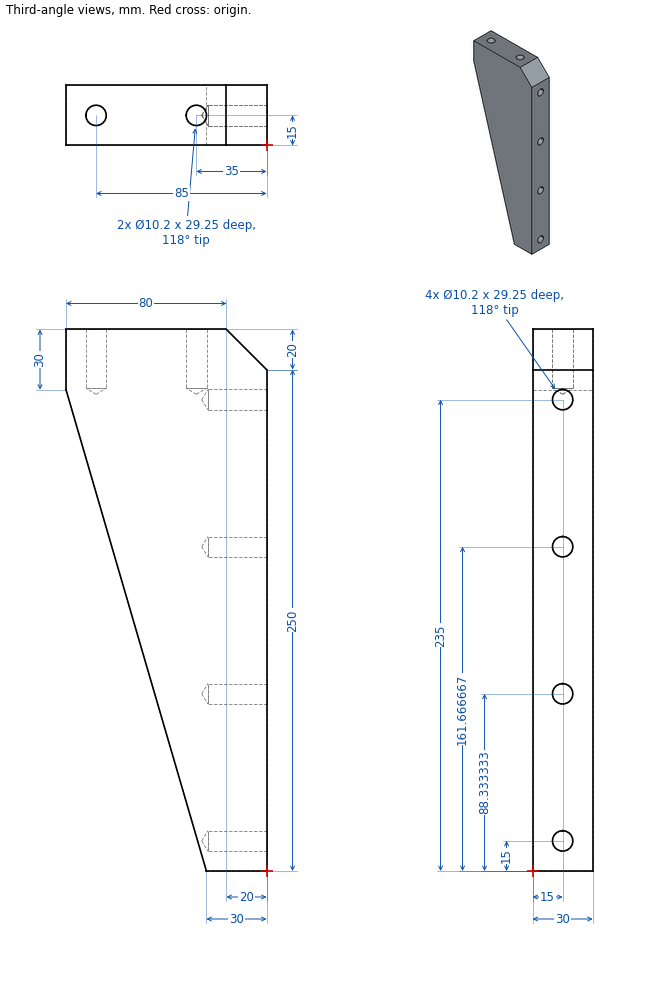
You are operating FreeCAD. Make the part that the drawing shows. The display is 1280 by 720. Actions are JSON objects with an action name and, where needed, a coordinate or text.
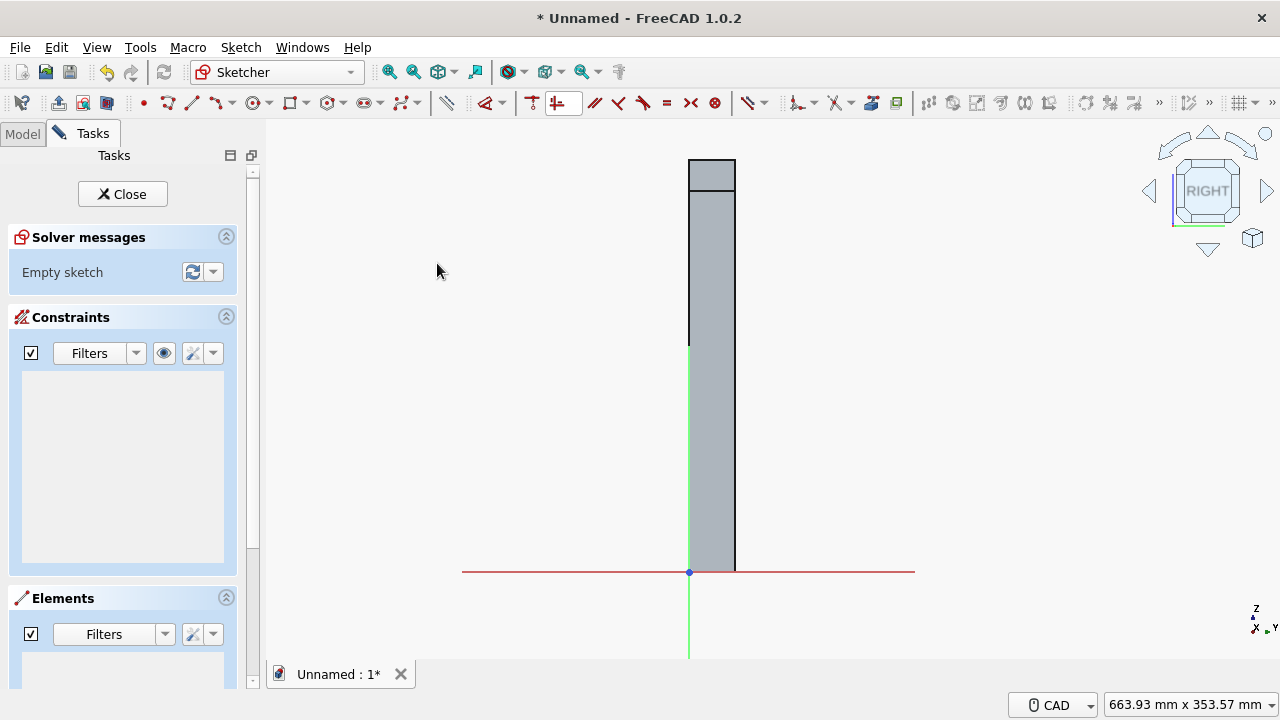
{"action": "key", "text": "g c"}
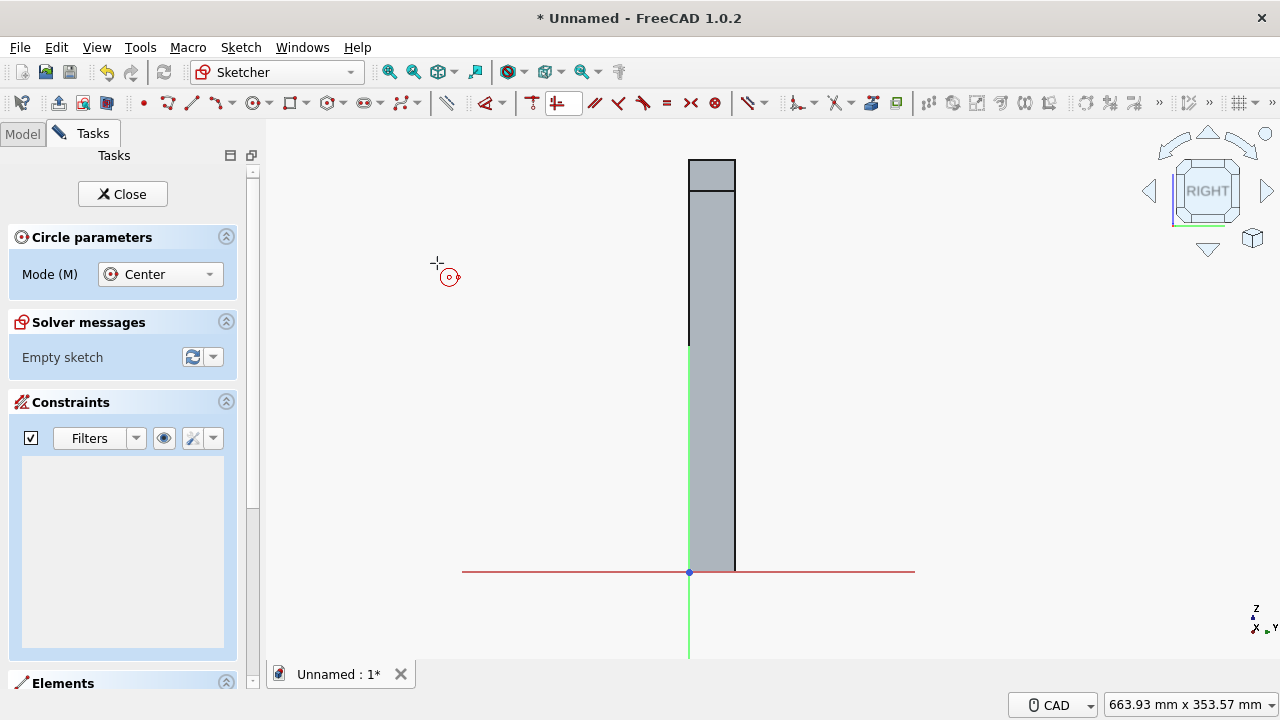
{"action": "scroll", "coordinate": [712, 213], "scroll_direction": "up", "scroll_amount": 6}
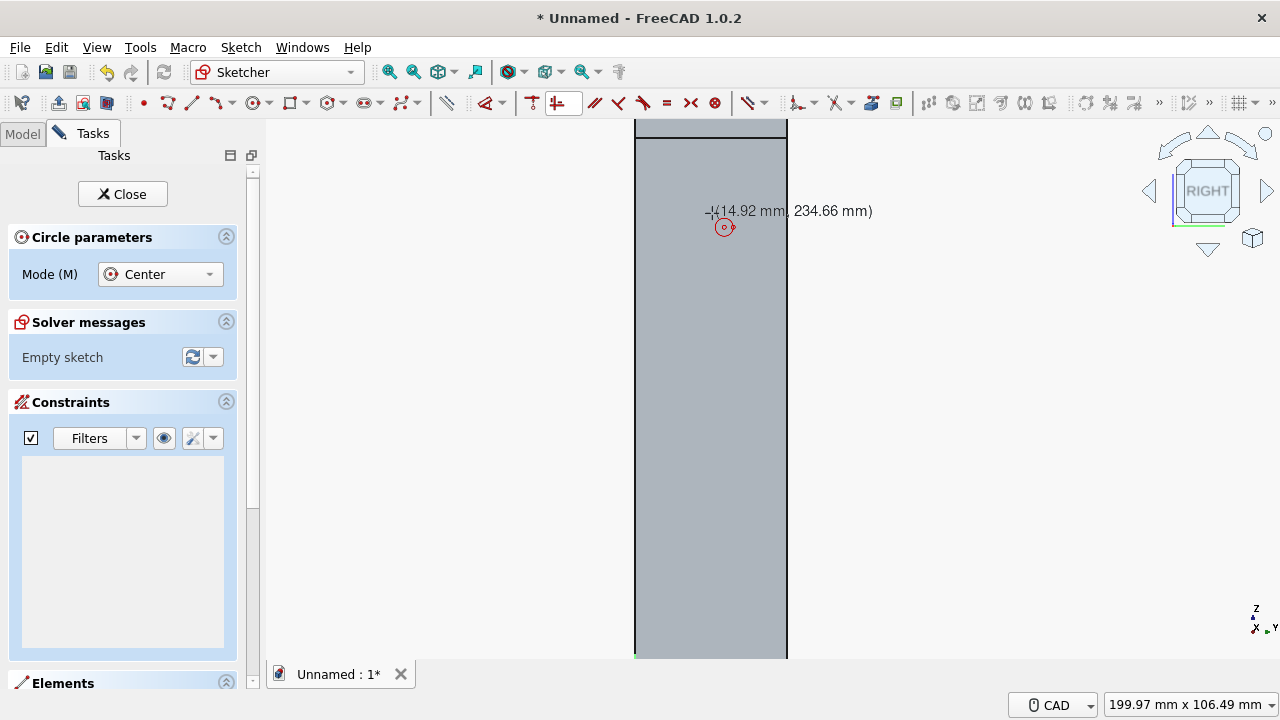
{"action": "left_click", "coordinate": [711, 214]}
{"action": "left_click", "coordinate": [730, 196]}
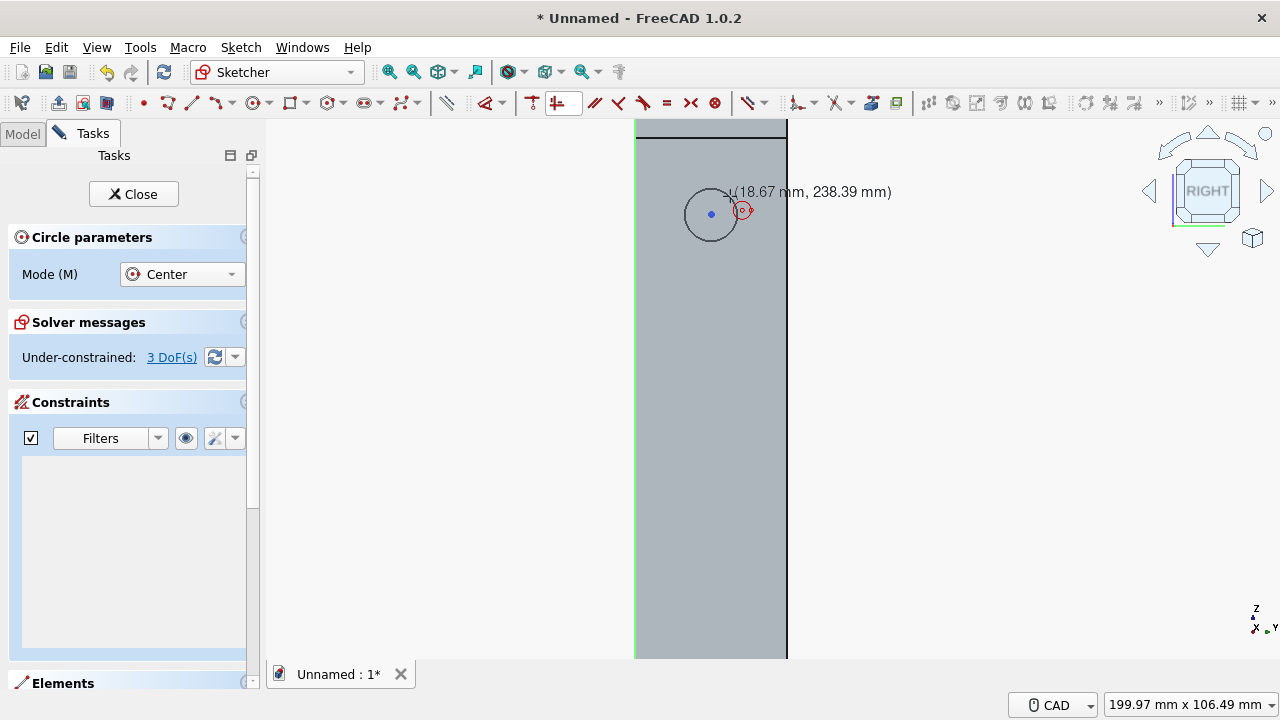
{"action": "scroll", "coordinate": [712, 213], "scroll_direction": "down", "scroll_amount": 6}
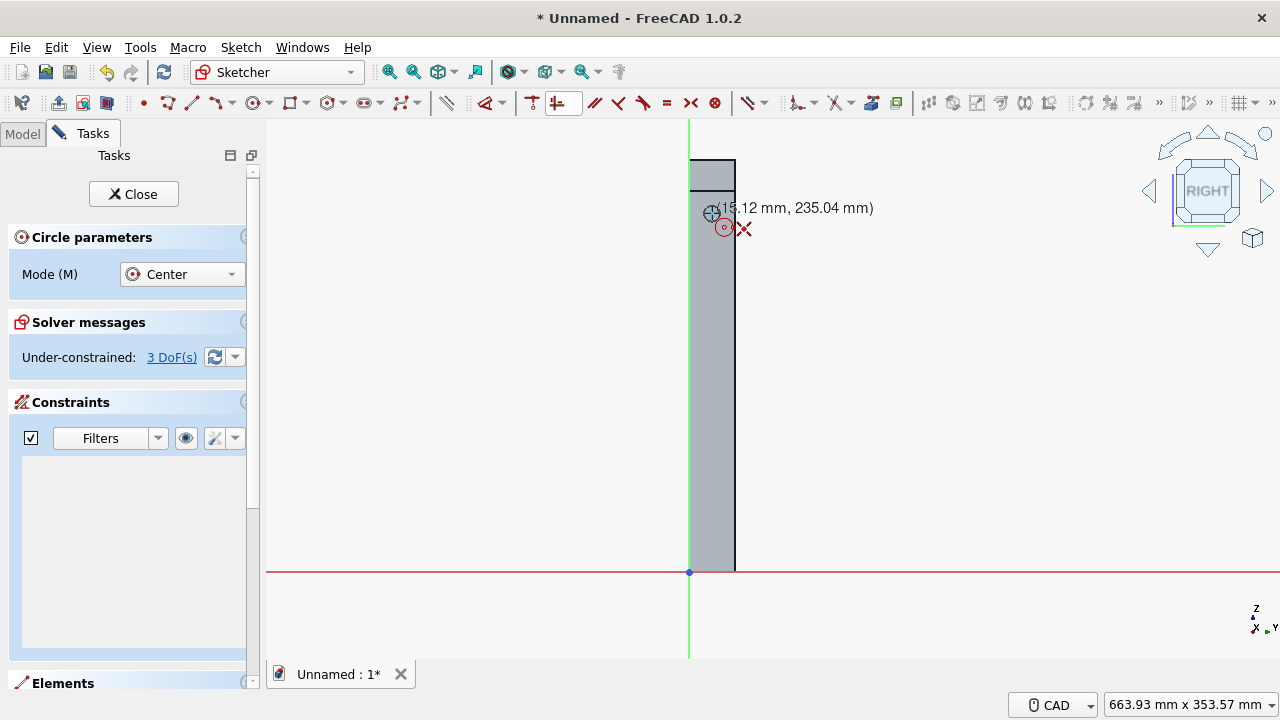
{"action": "scroll", "coordinate": [712, 549], "scroll_direction": "up", "scroll_amount": 6}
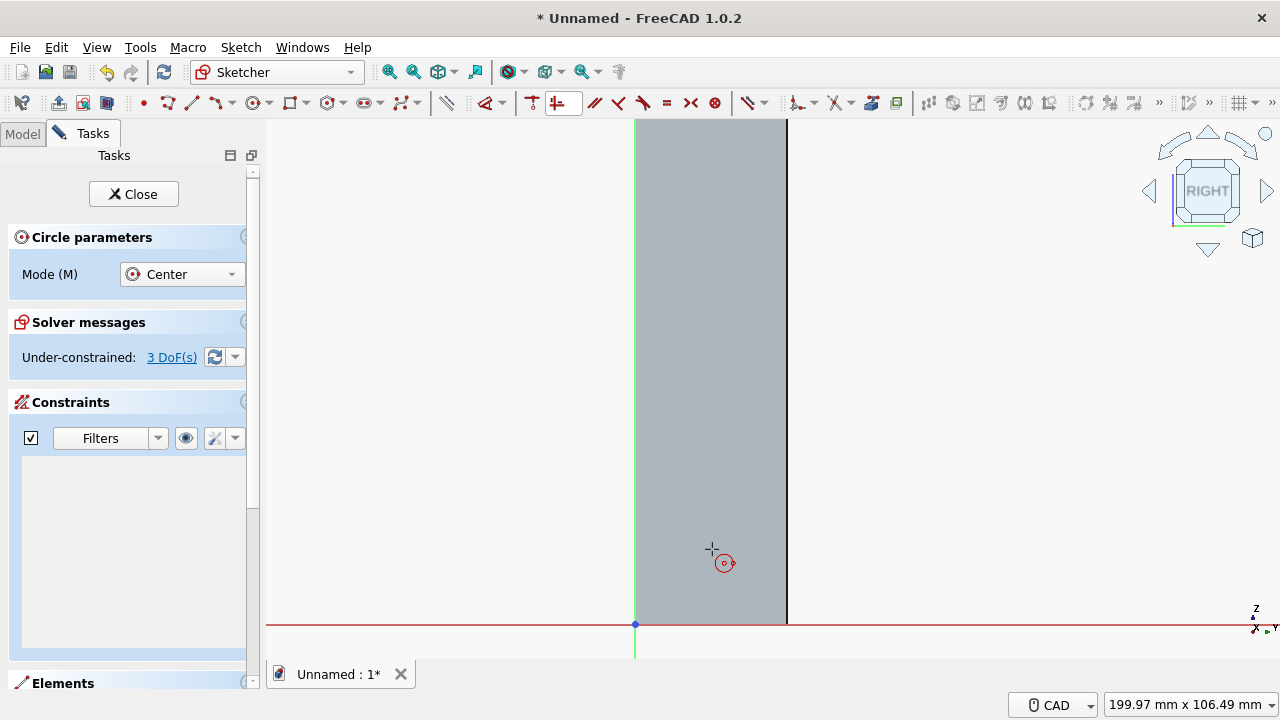
{"action": "left_click", "coordinate": [711, 549]}
{"action": "left_click", "coordinate": [730, 530]}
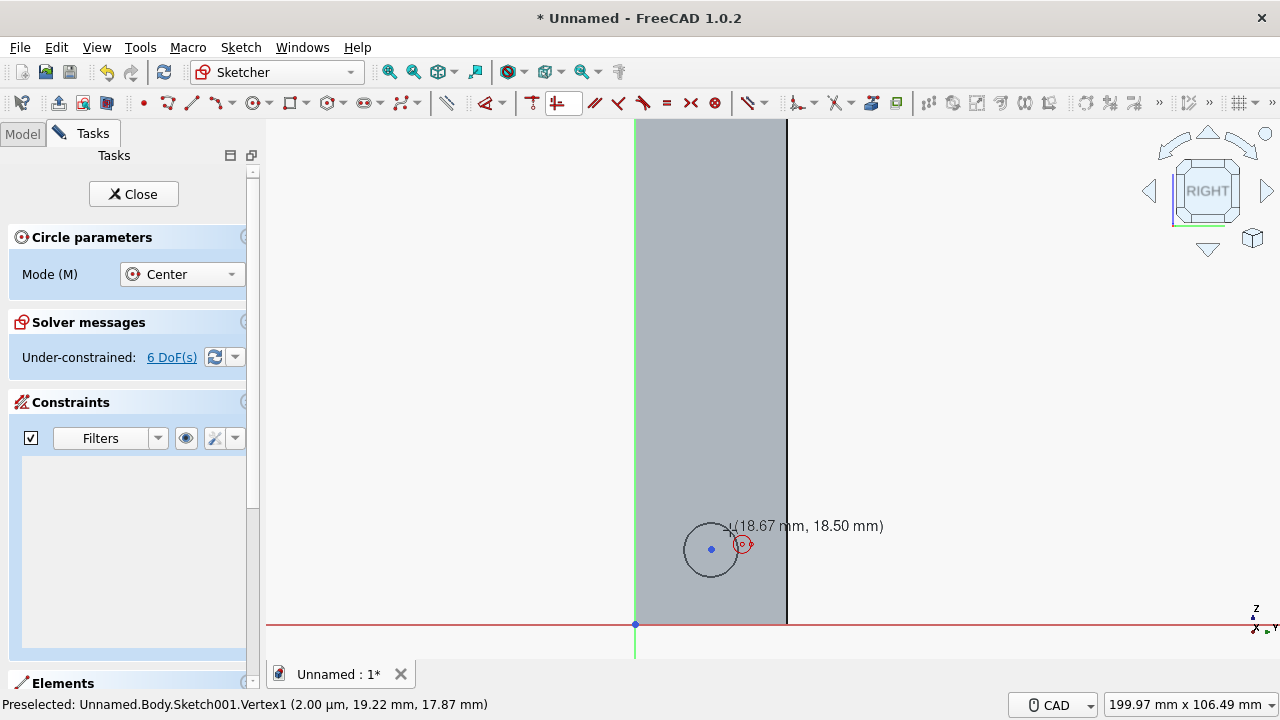
{"action": "left_click", "coordinate": [711, 177]}
{"action": "left_click", "coordinate": [730, 159]}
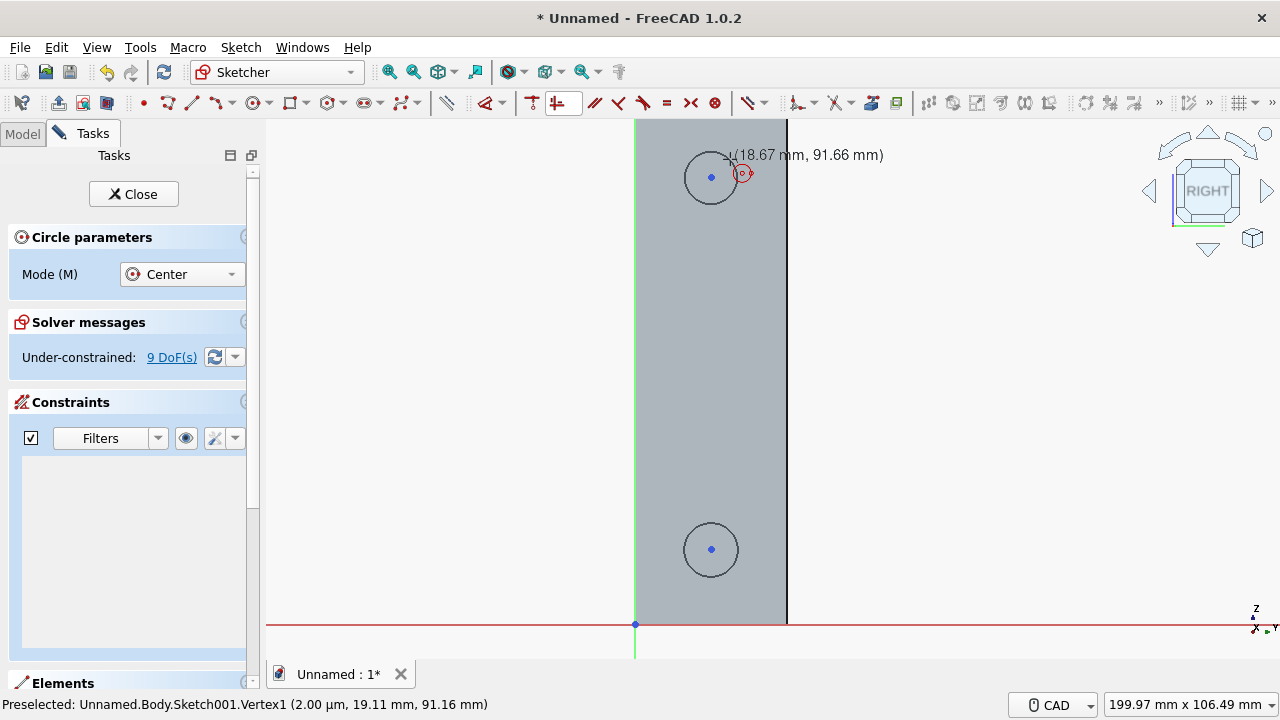
{"action": "scroll", "coordinate": [712, 550], "scroll_direction": "down", "scroll_amount": 6}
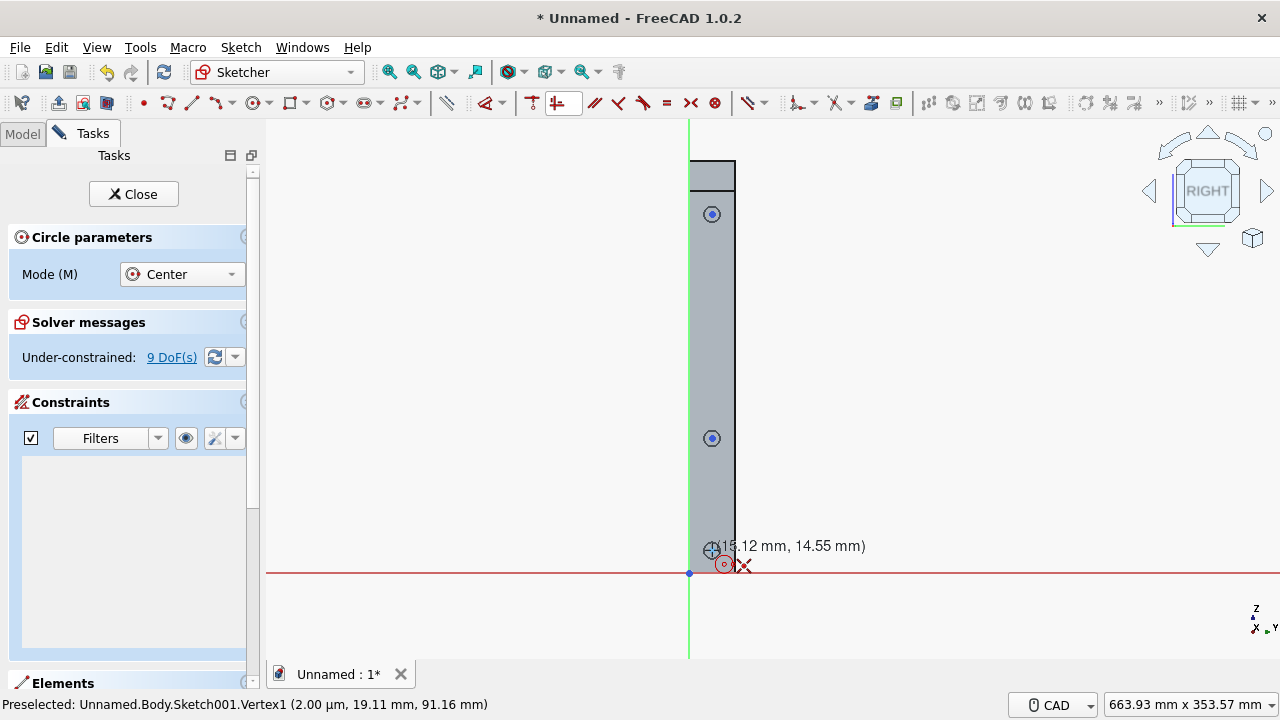
{"action": "scroll", "coordinate": [712, 326], "scroll_direction": "up", "scroll_amount": 6}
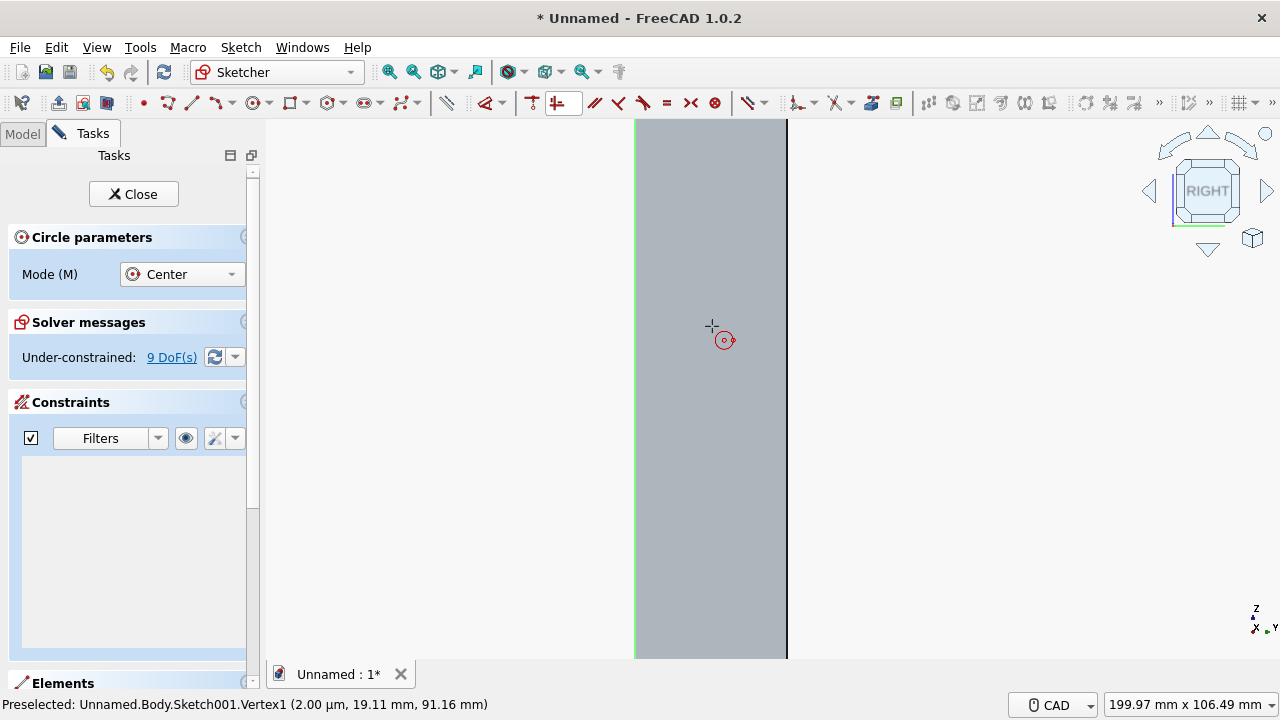
{"action": "left_click", "coordinate": [711, 326]}
{"action": "left_click", "coordinate": [730, 307]}
{"action": "key", "text": "Escape"}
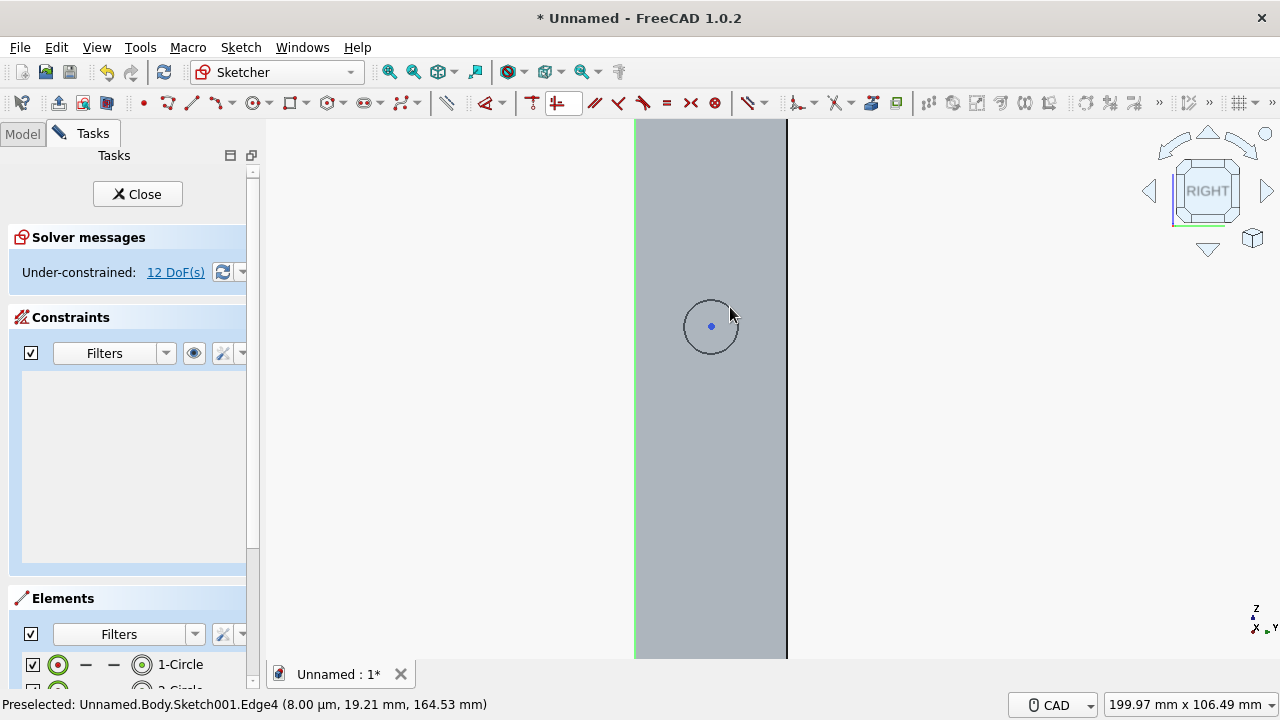
{"action": "scroll", "coordinate": [712, 325], "scroll_direction": "down", "scroll_amount": 6}